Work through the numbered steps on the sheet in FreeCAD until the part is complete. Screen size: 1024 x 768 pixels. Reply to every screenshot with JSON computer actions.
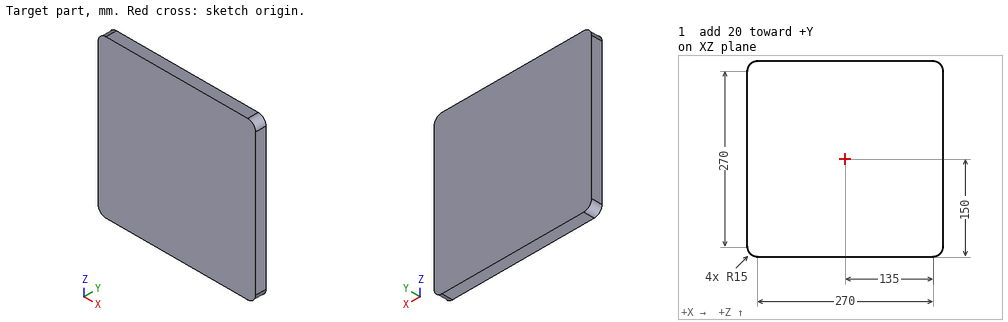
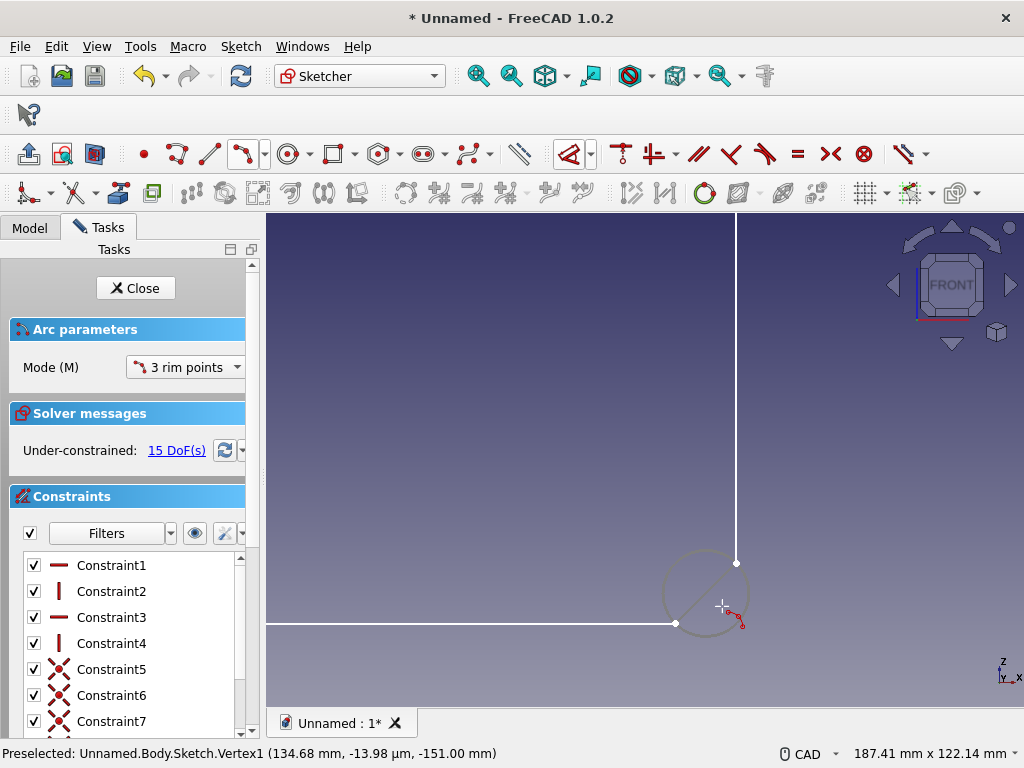
{"action": "left_click", "coordinate": [720, 602]}
{"action": "key", "text": "Escape"}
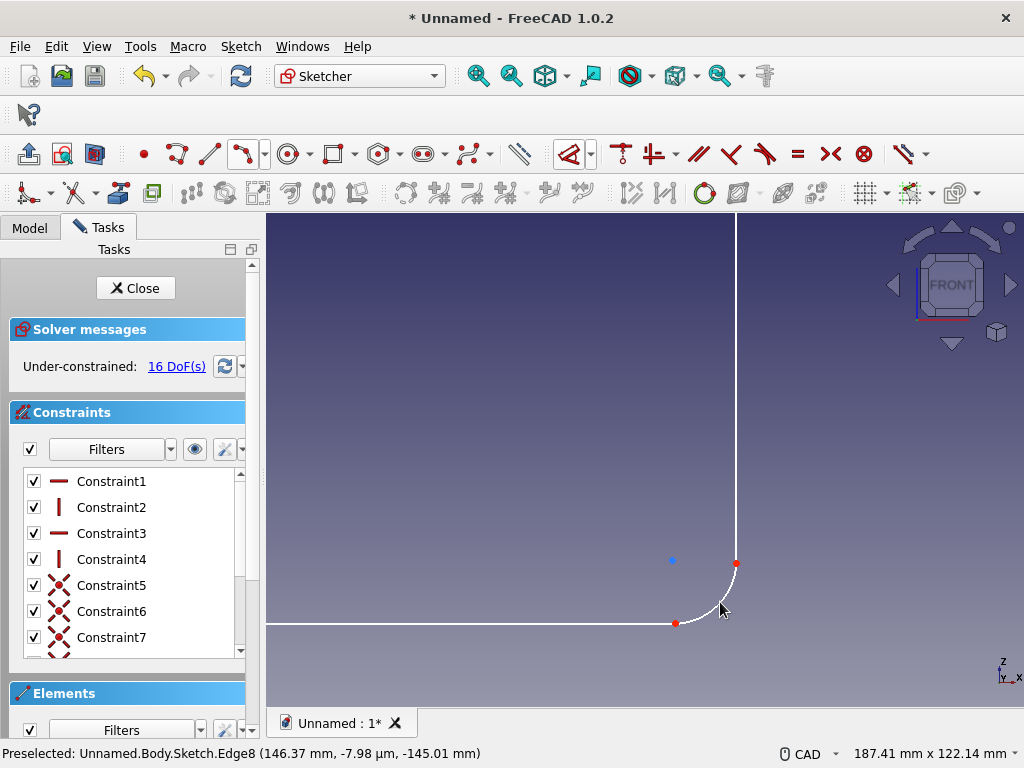
{"action": "scroll", "coordinate": [722, 606], "scroll_direction": "down", "scroll_amount": 7}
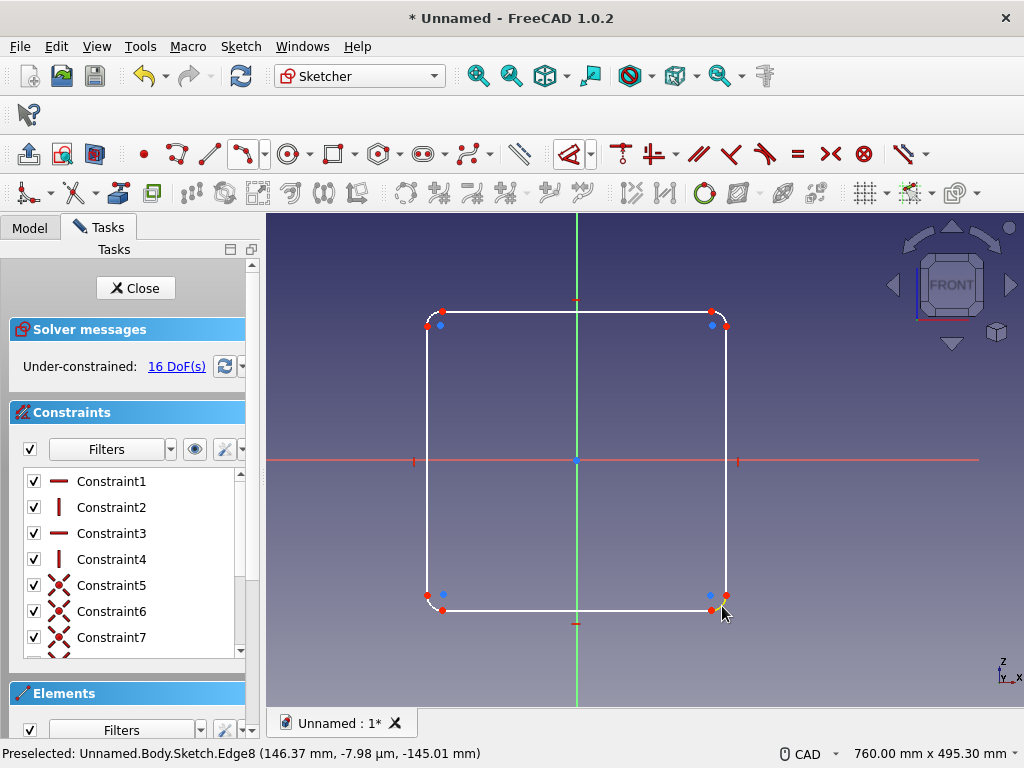
{"action": "left_click", "coordinate": [630, 611]}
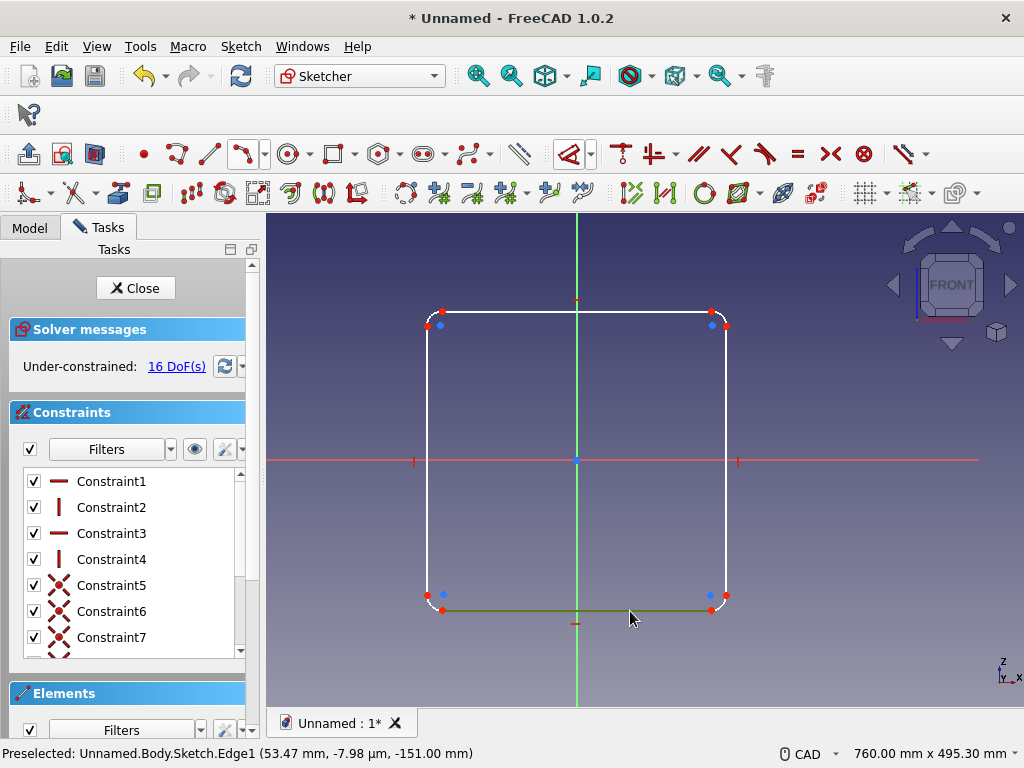
{"action": "scroll", "coordinate": [432, 606], "scroll_direction": "up", "scroll_amount": 2}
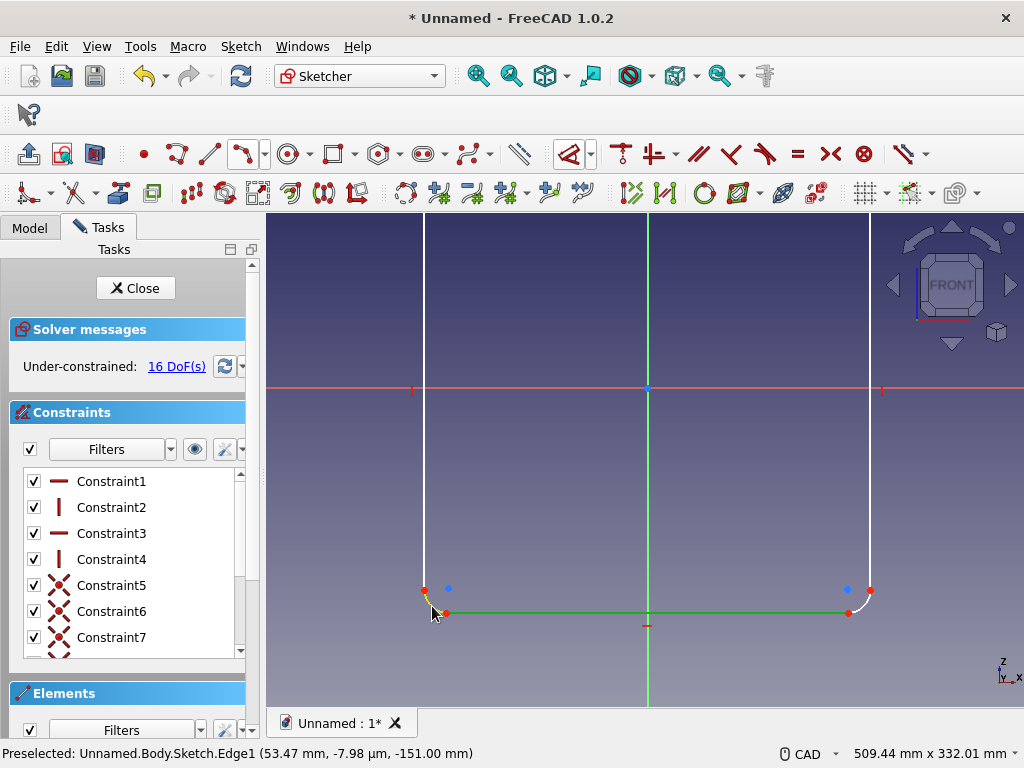
{"action": "left_click", "coordinate": [432, 606]}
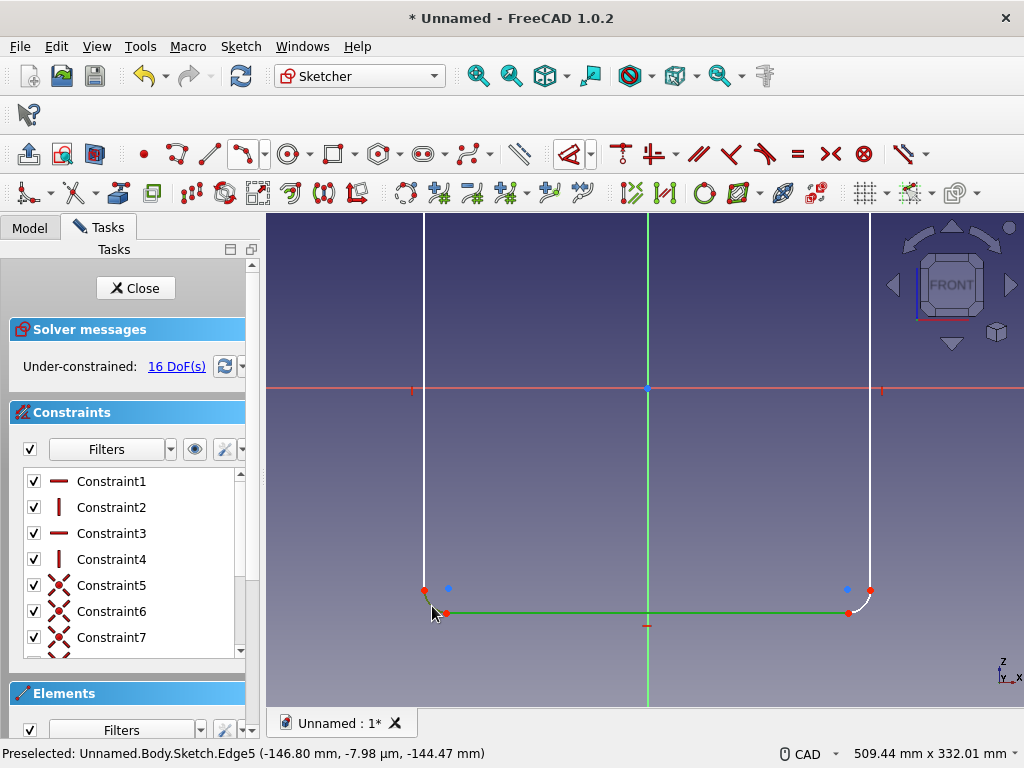
{"action": "left_click", "coordinate": [765, 154]}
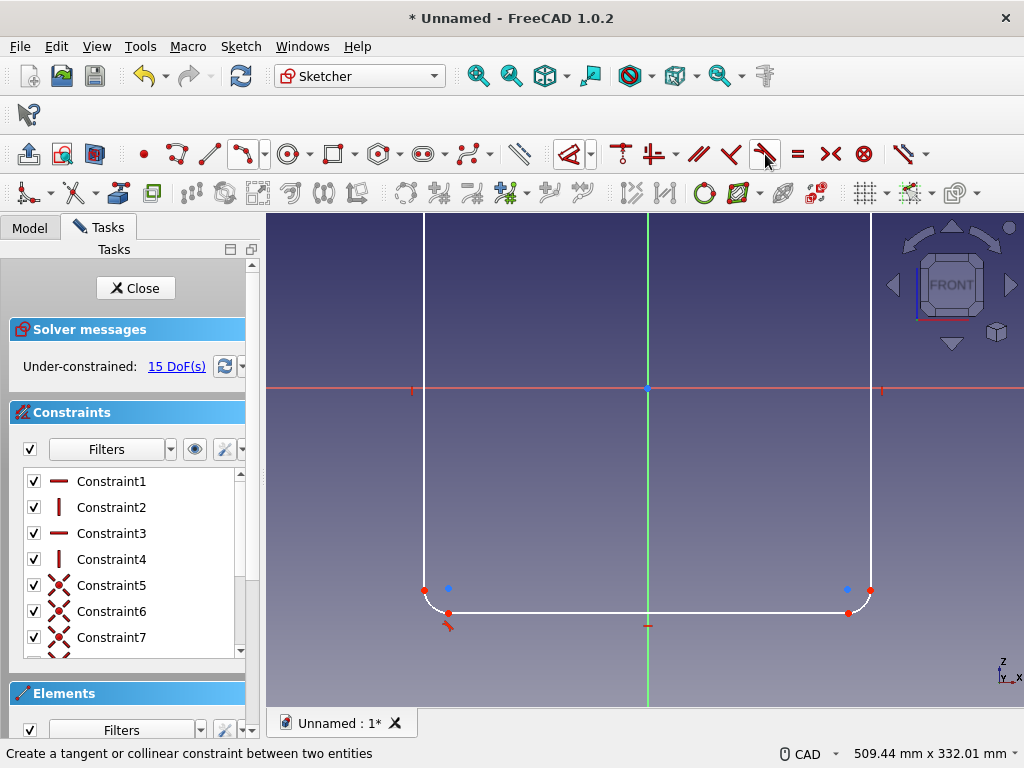
{"action": "left_click", "coordinate": [728, 613]}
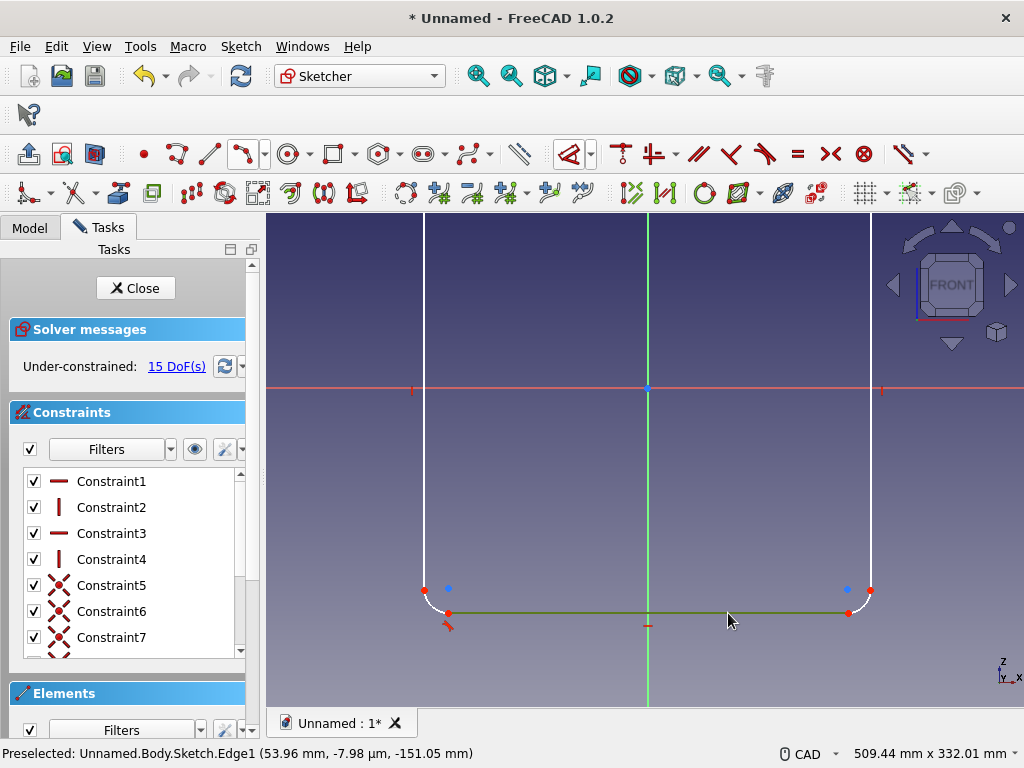
{"action": "scroll", "coordinate": [858, 610], "scroll_direction": "up", "scroll_amount": 2}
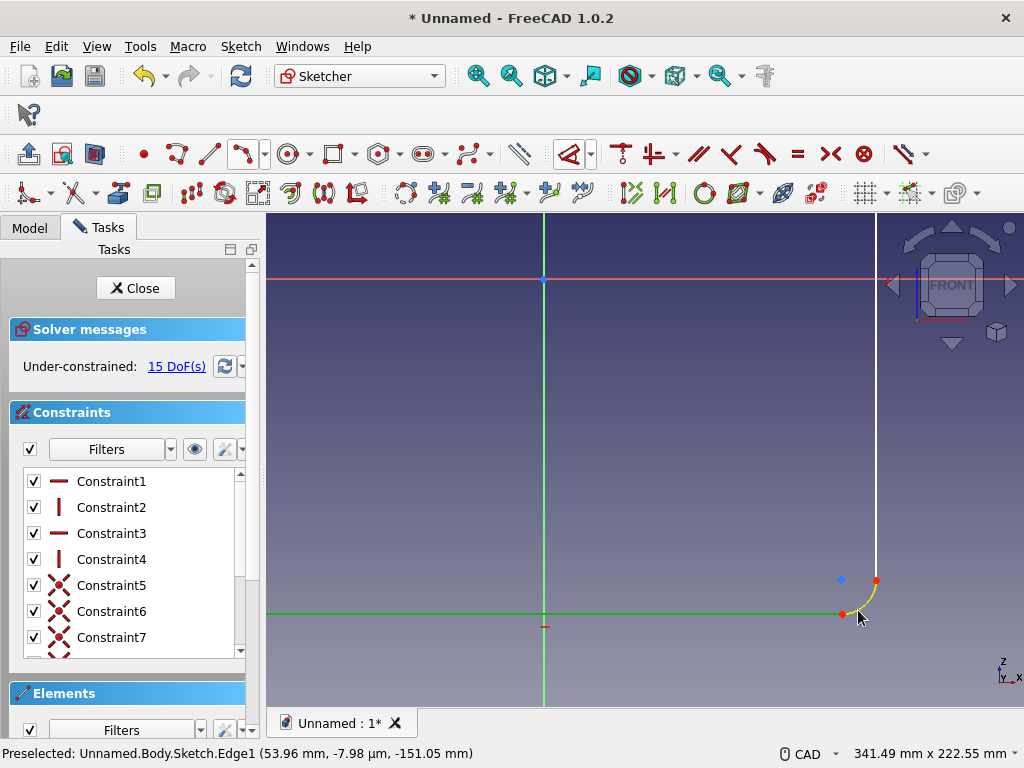
{"action": "left_click", "coordinate": [858, 610]}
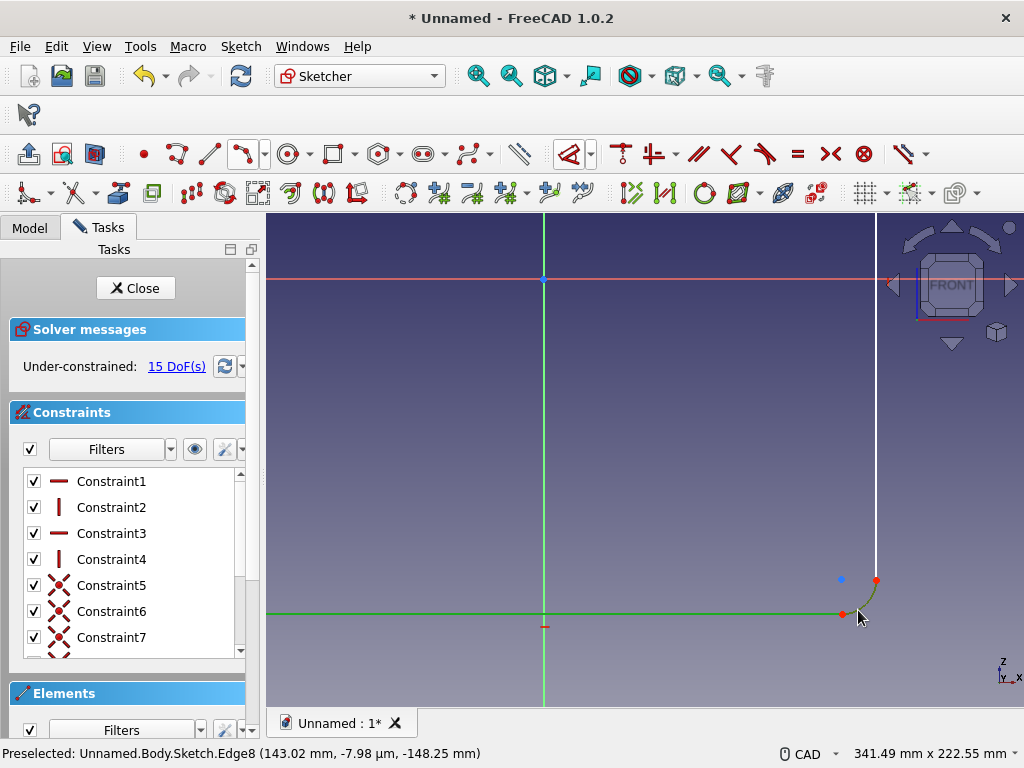
{"action": "left_click", "coordinate": [765, 154]}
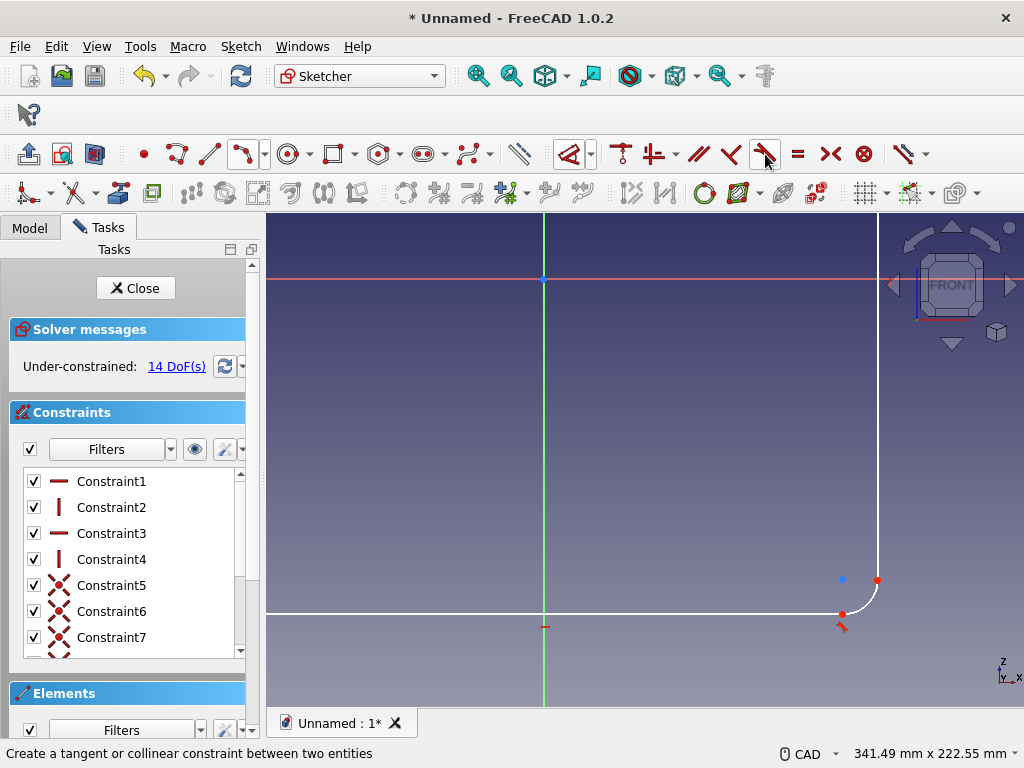
{"action": "scroll", "coordinate": [603, 608], "scroll_direction": "down", "scroll_amount": 4}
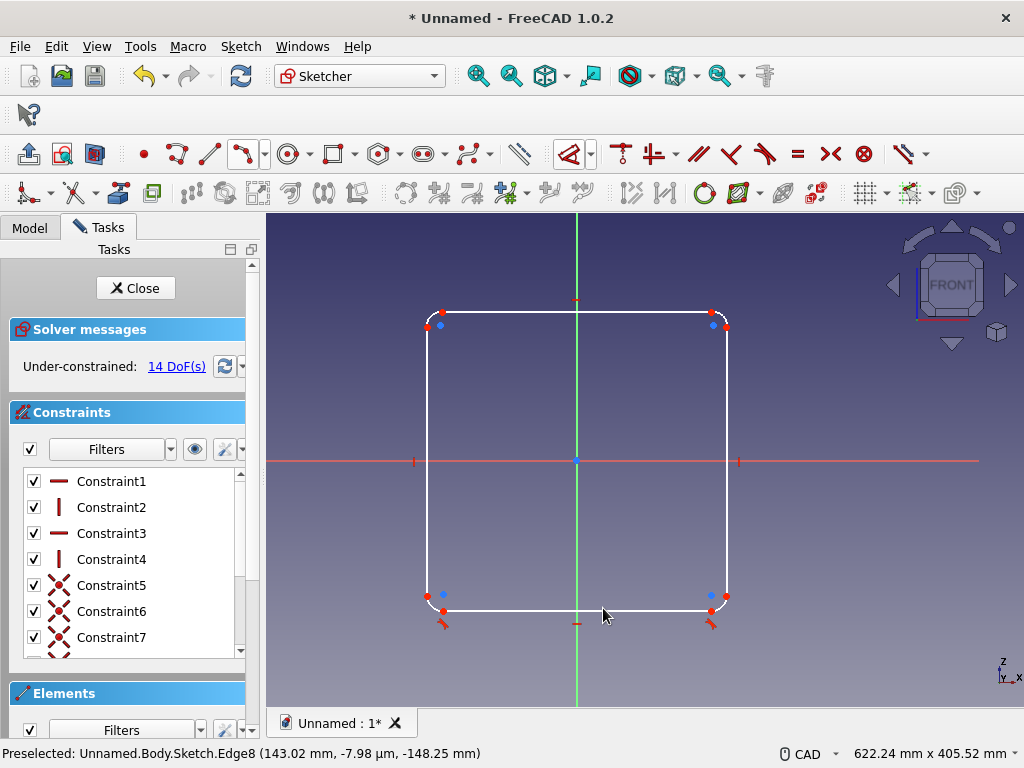
{"action": "left_click", "coordinate": [427, 516]}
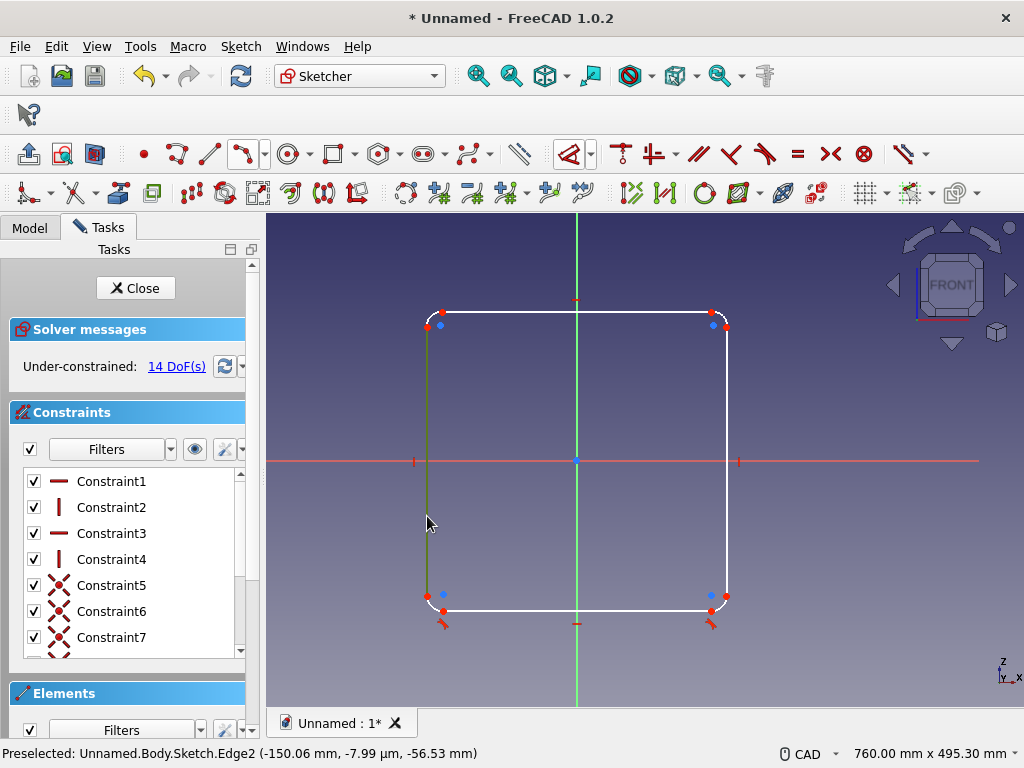
{"action": "left_click", "coordinate": [432, 607]}